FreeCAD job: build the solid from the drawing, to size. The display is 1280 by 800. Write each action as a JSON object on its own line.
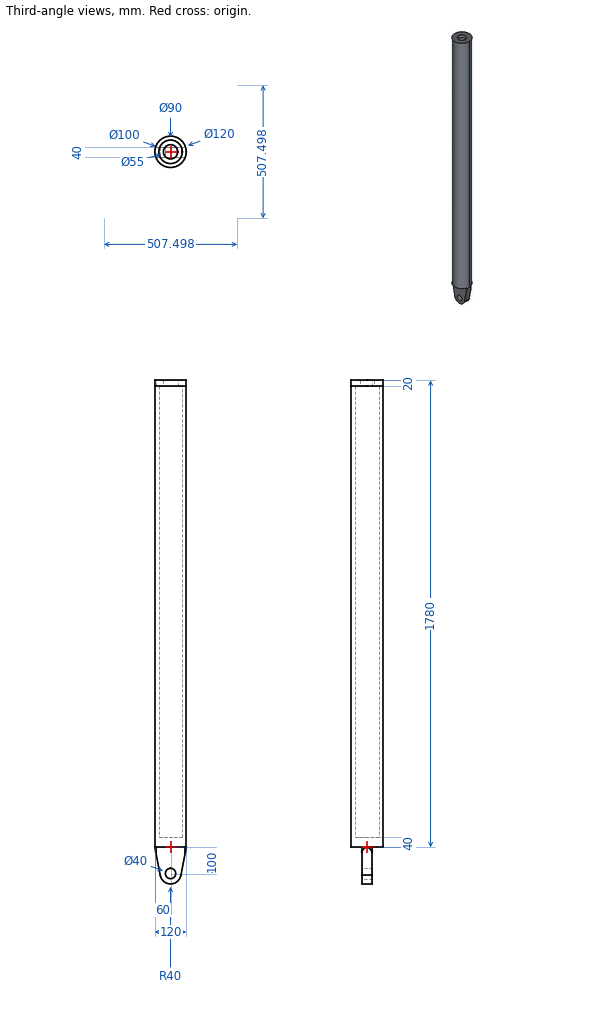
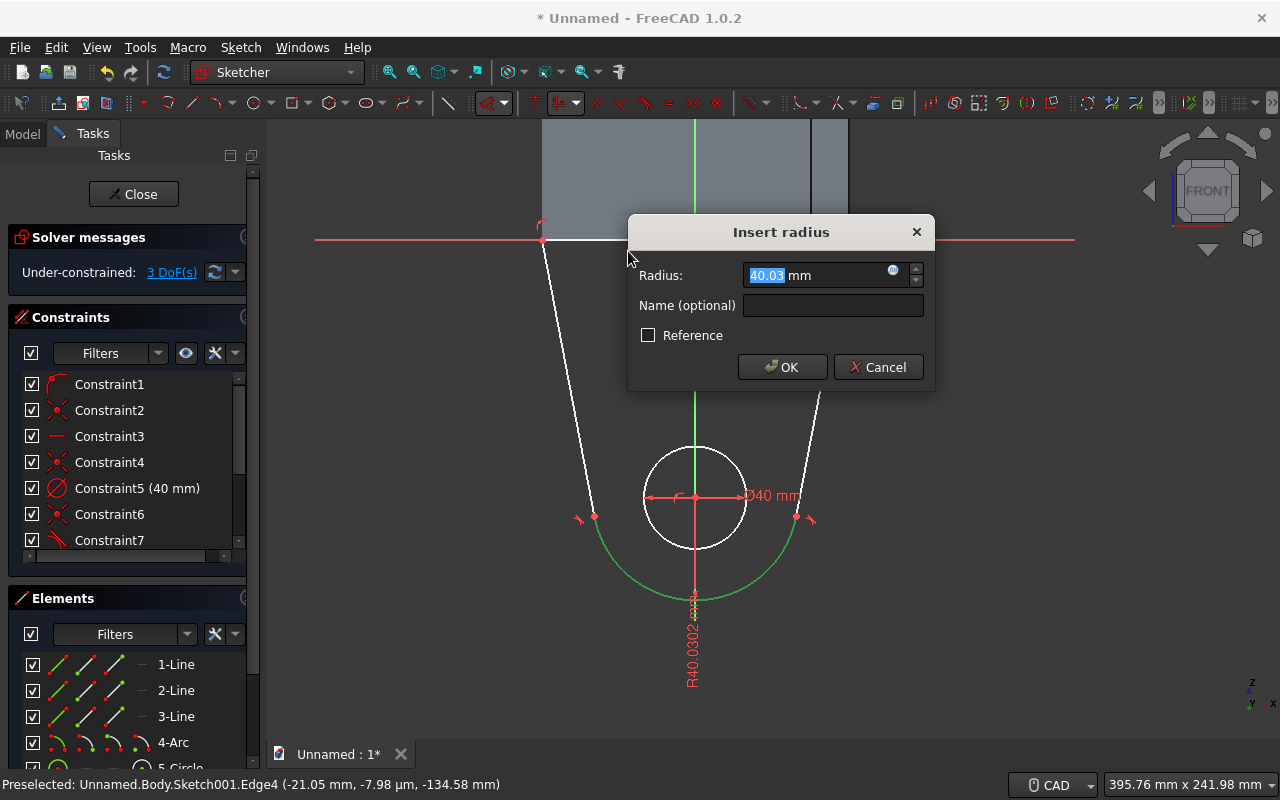
{"action": "type", "text": "40"}
{"action": "key", "text": "Return"}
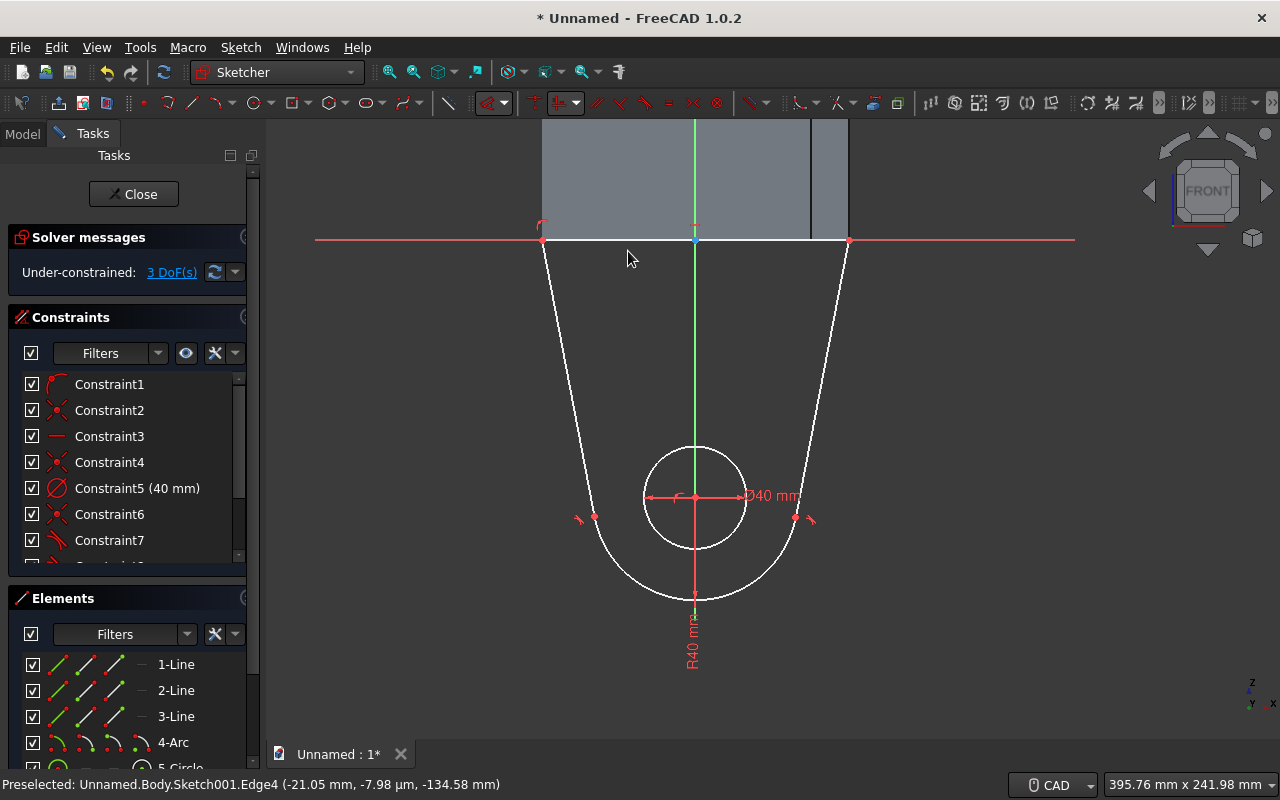
{"action": "left_click", "coordinate": [634, 240]}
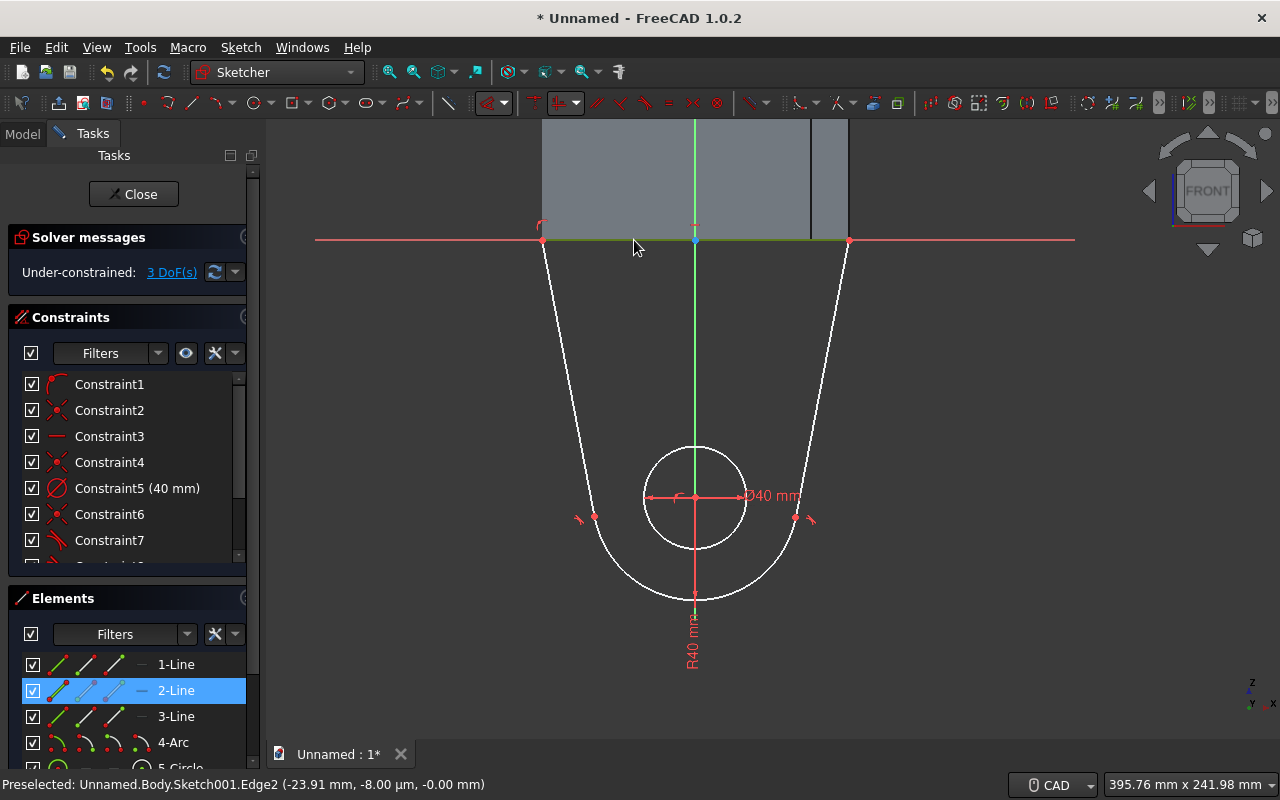
{"action": "key", "text": "l"}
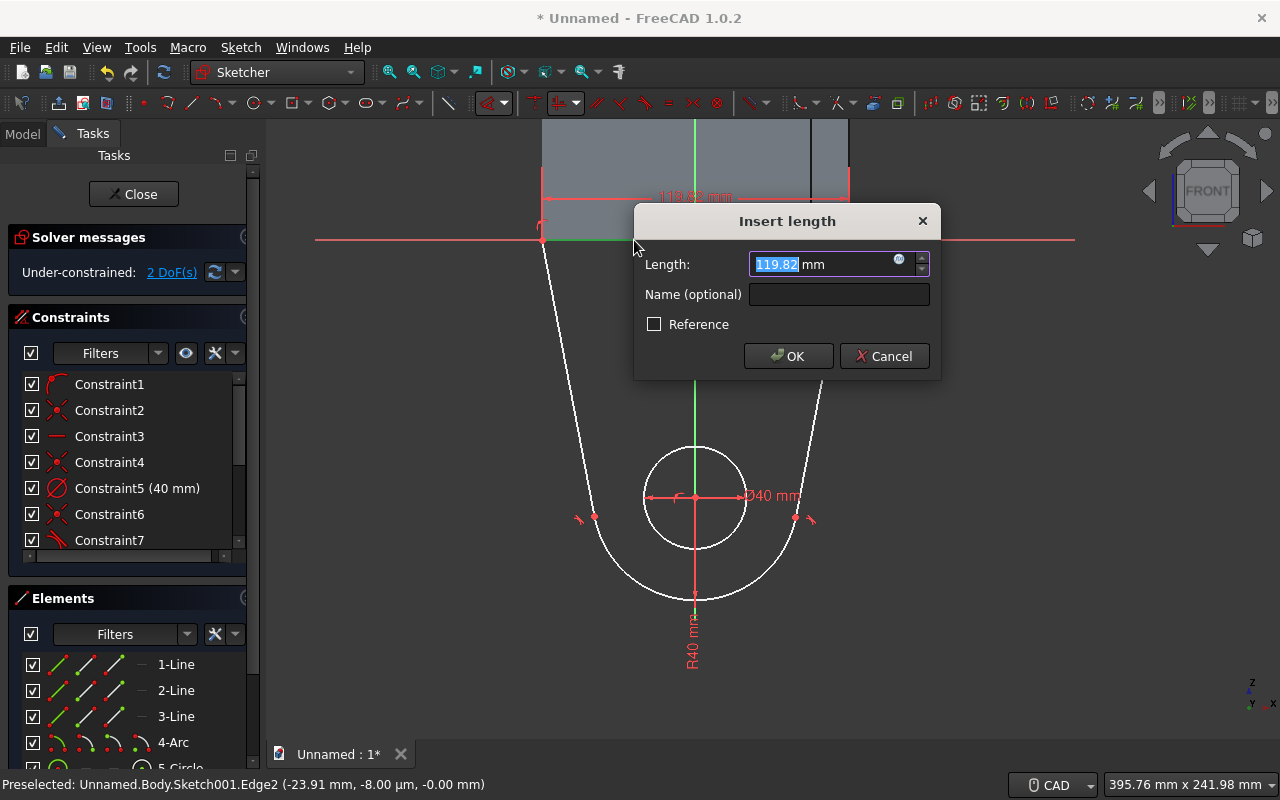
{"action": "type", "text": "120"}
{"action": "key", "text": "Return"}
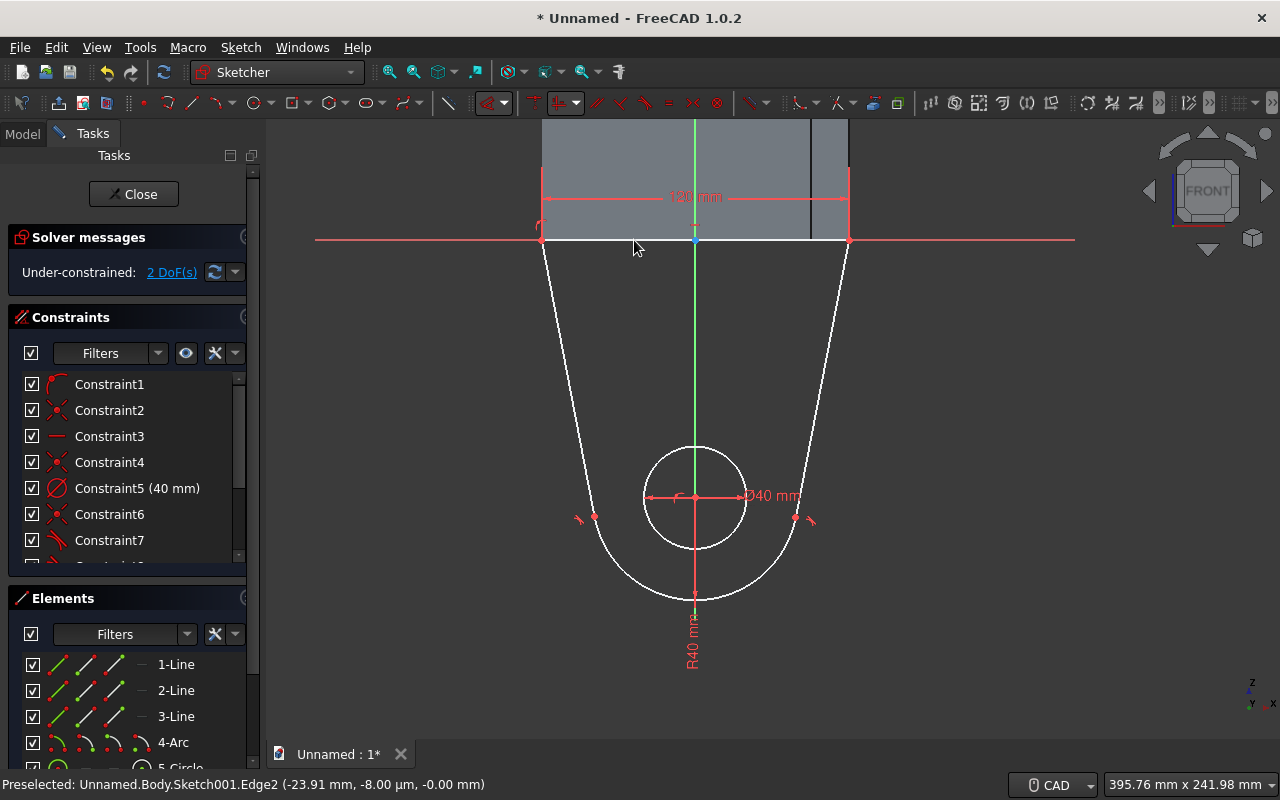
{"action": "left_click", "coordinate": [542, 240]}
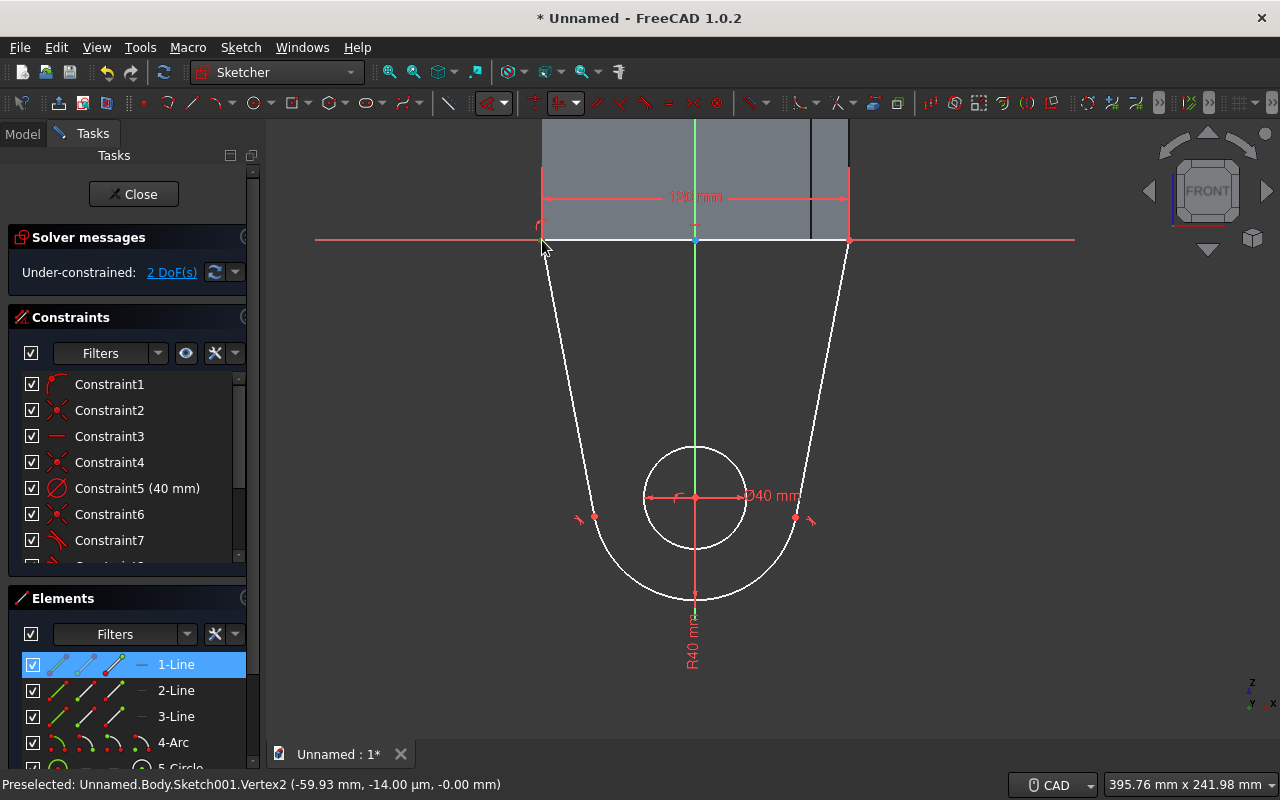
{"action": "key", "text": "l"}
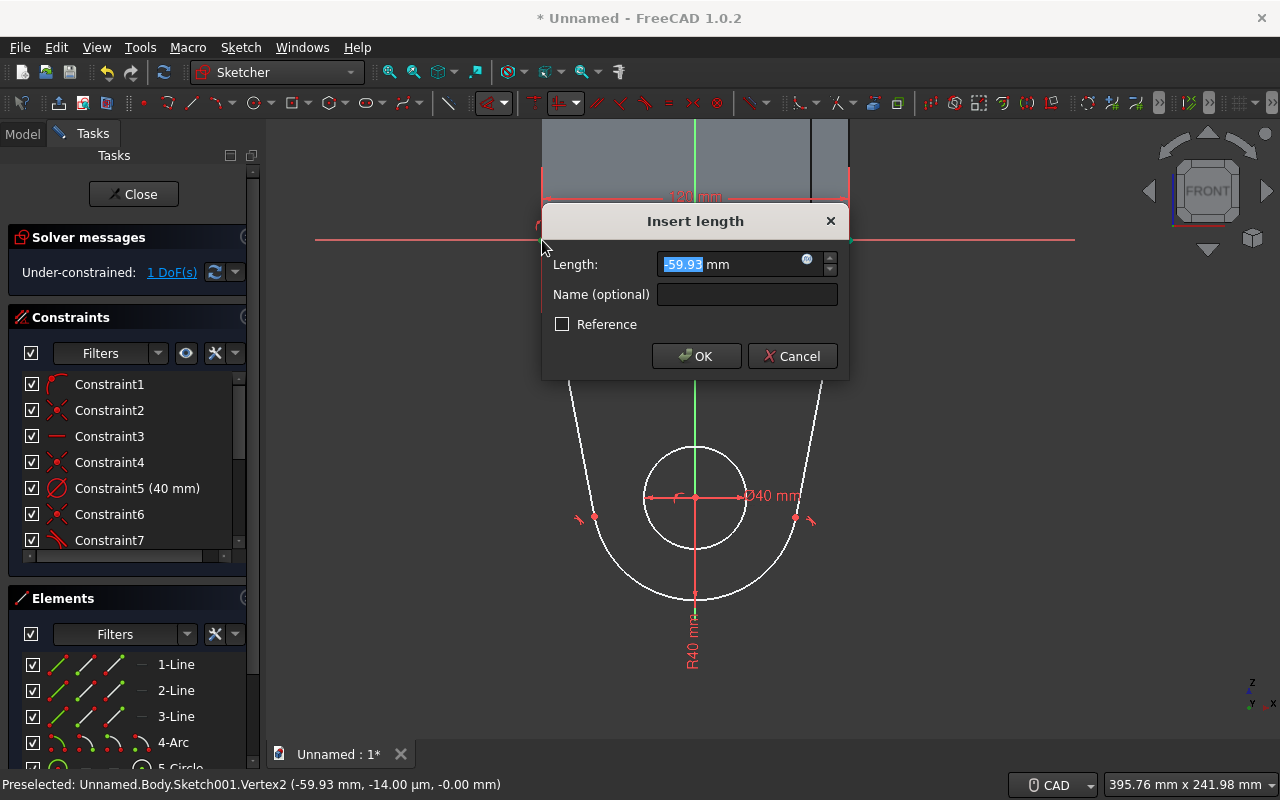
{"action": "type", "text": "-60"}
{"action": "key", "text": "Return"}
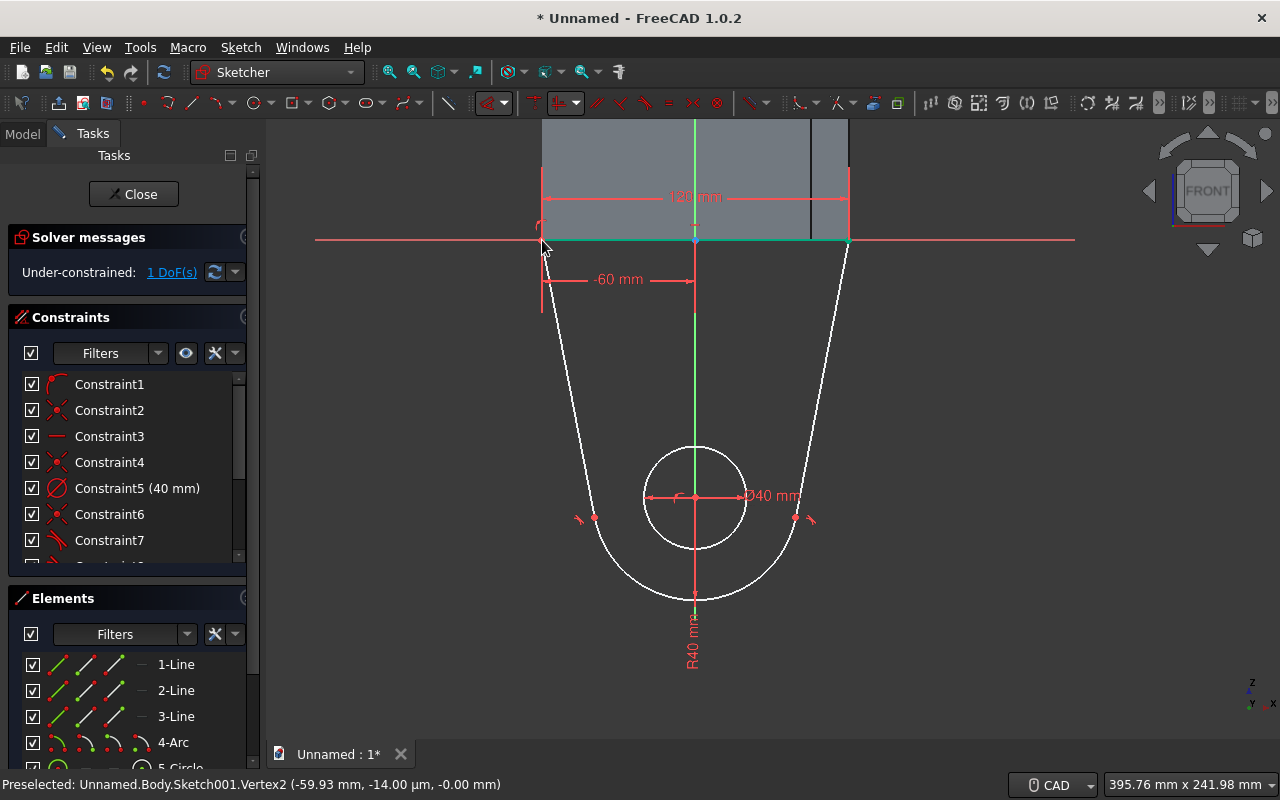
{"action": "left_click", "coordinate": [695, 498]}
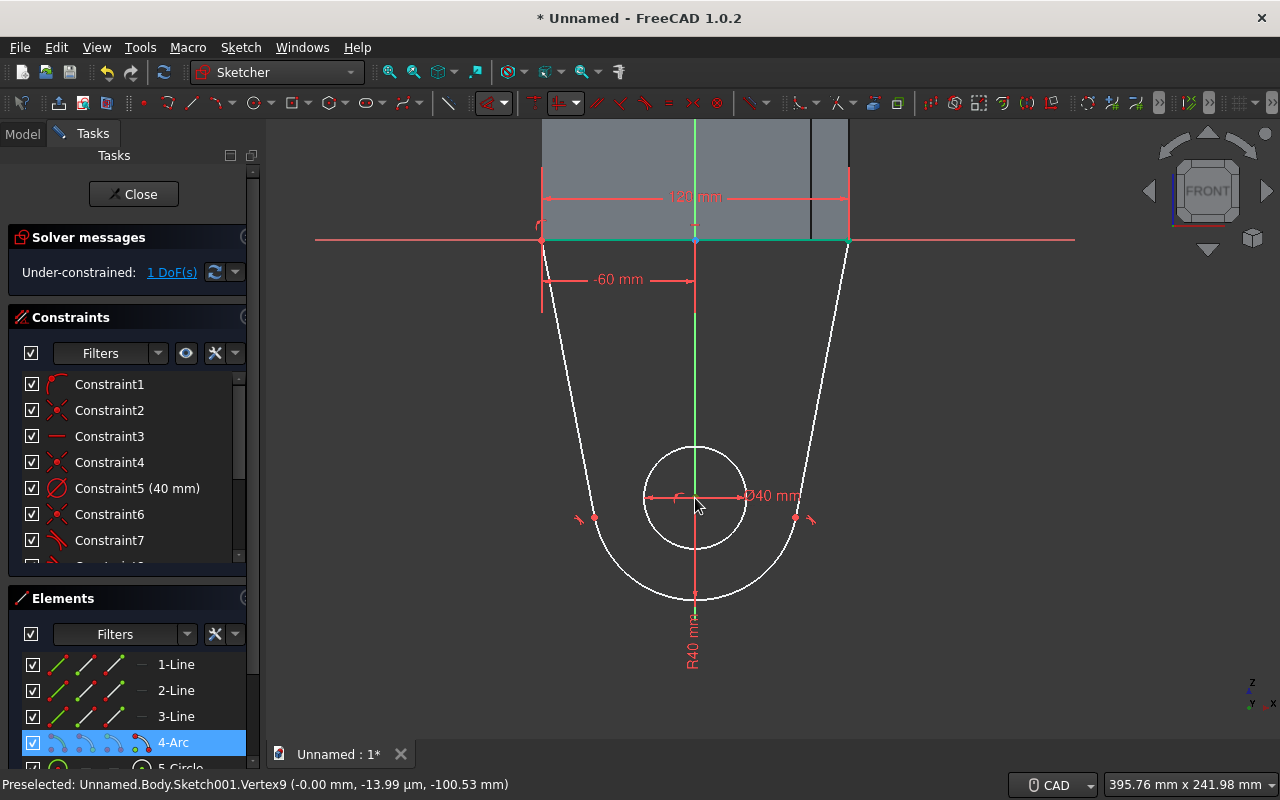
{"action": "key", "text": "i"}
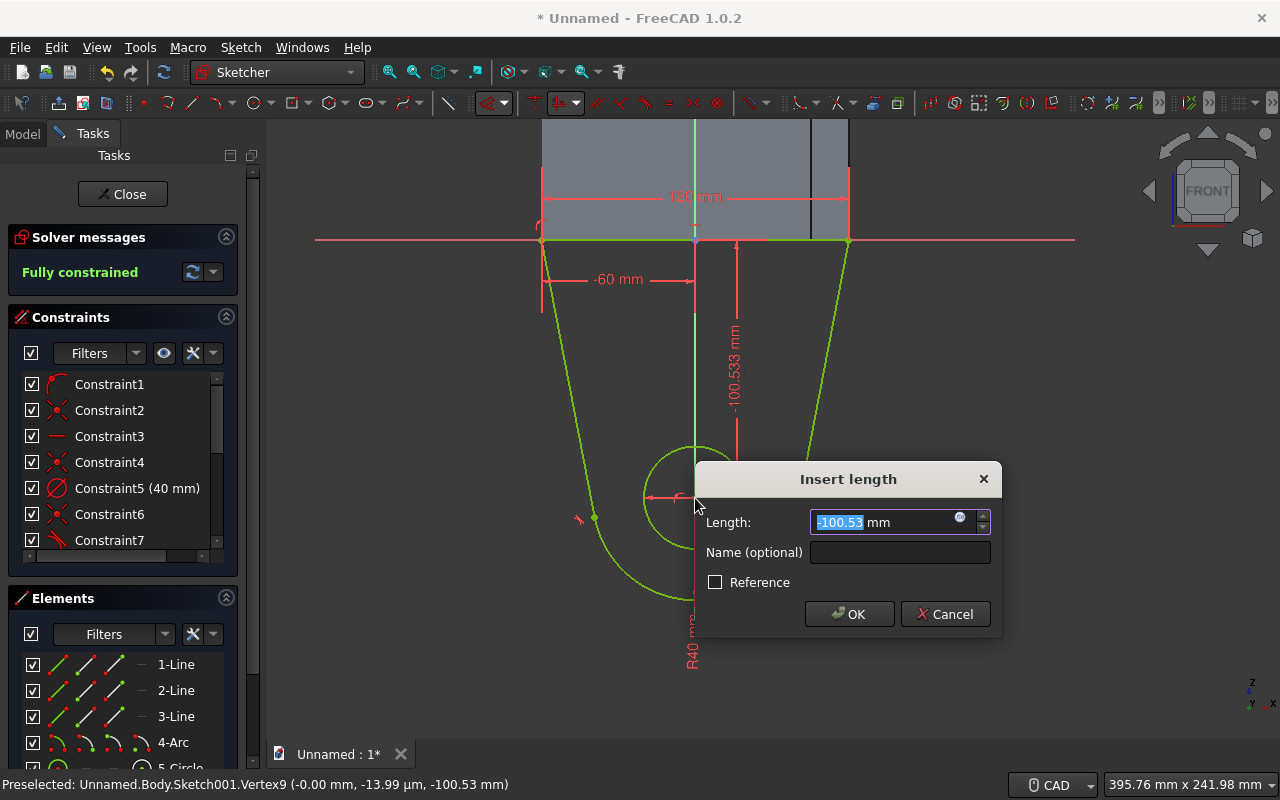
{"action": "type", "text": "-100"}
{"action": "key", "text": "Return"}